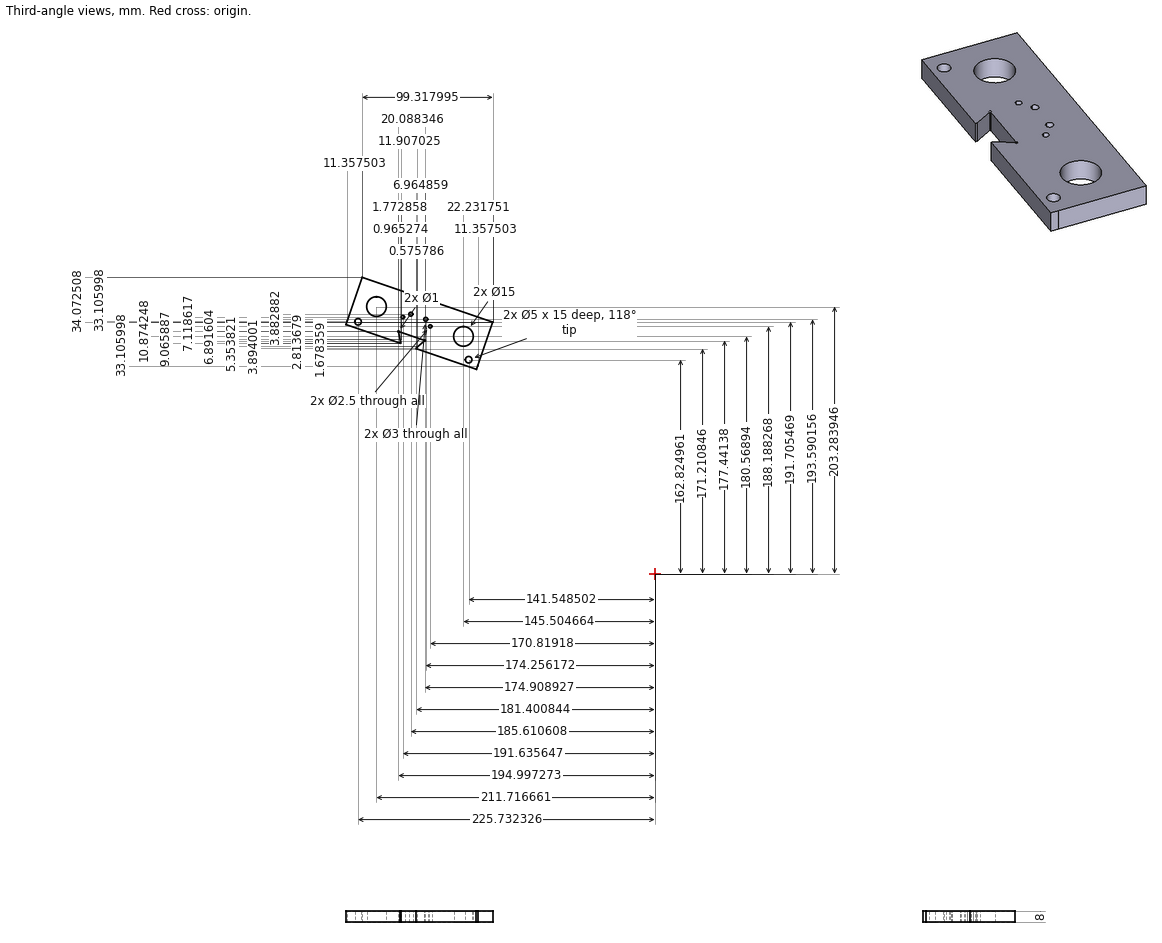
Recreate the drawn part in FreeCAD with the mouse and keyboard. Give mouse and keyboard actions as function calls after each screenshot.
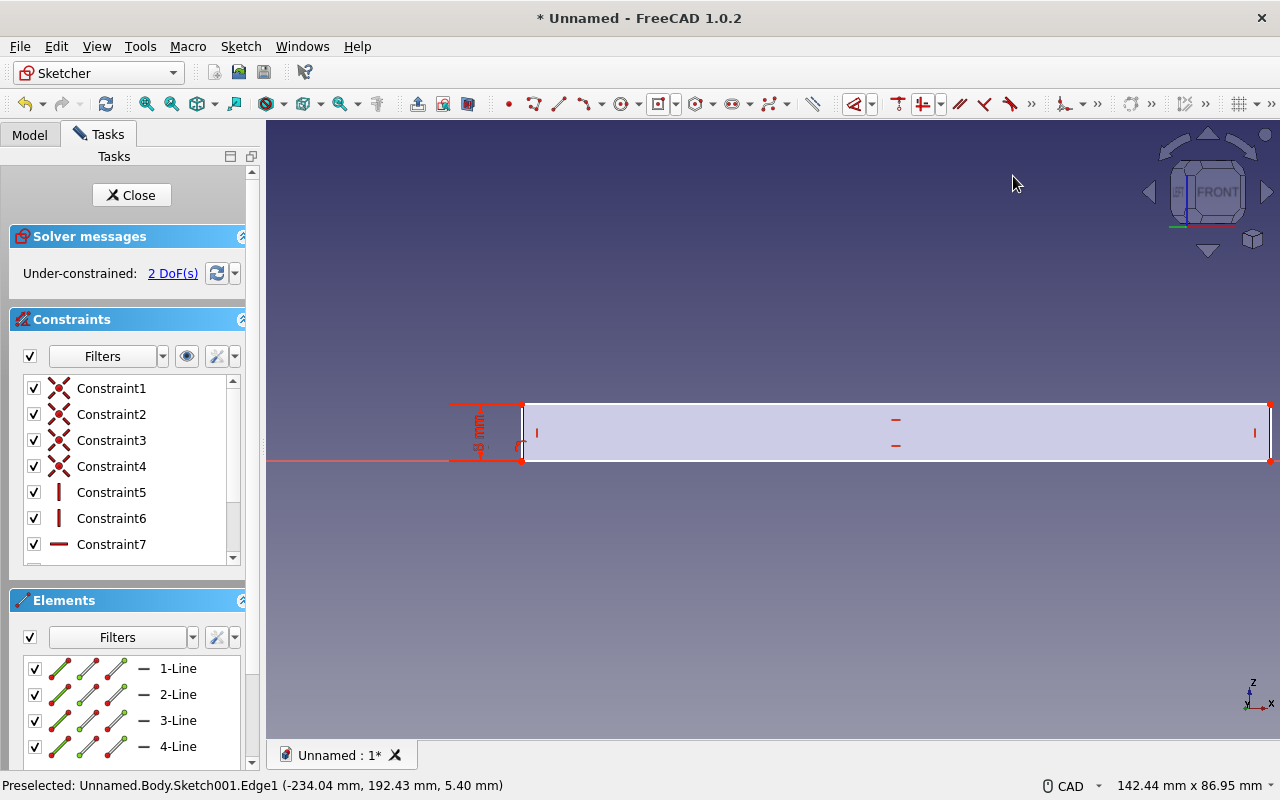
click(747, 461)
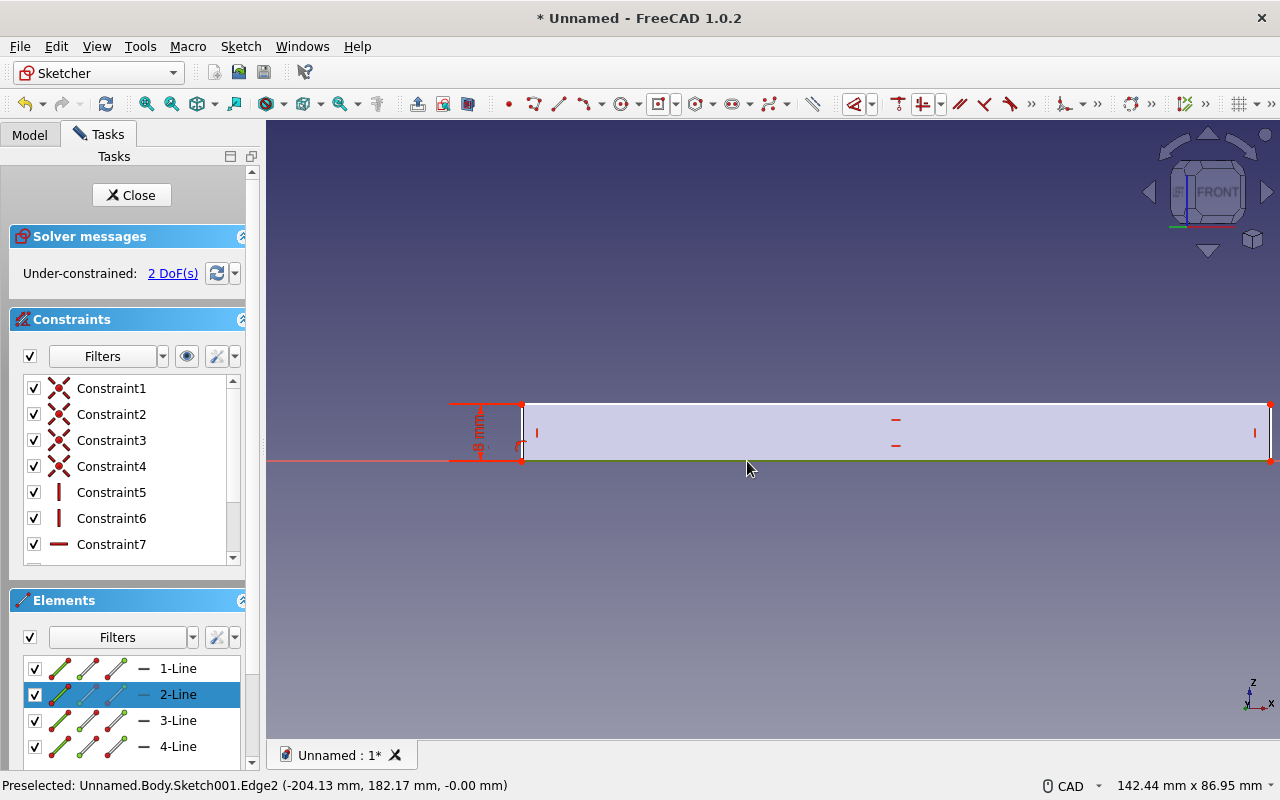
click(872, 104)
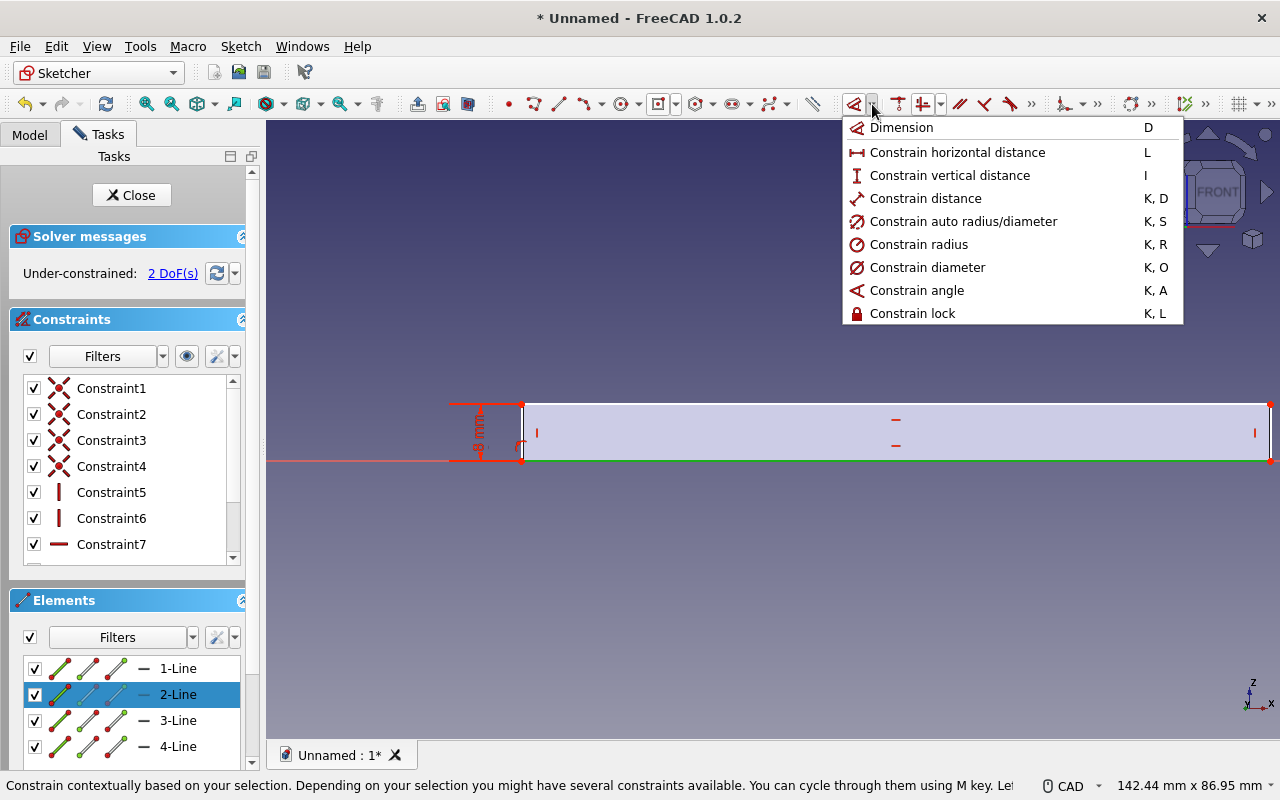
click(1013, 152)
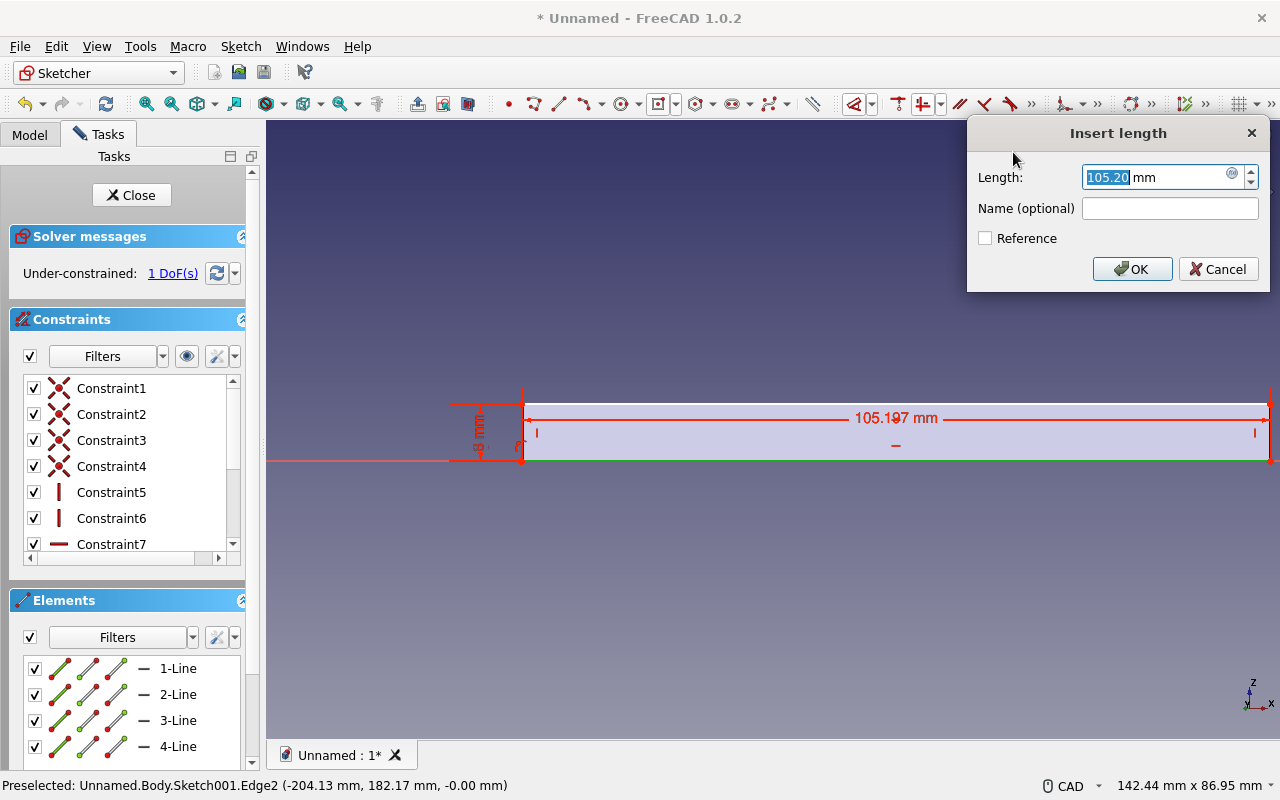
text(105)
key(Return)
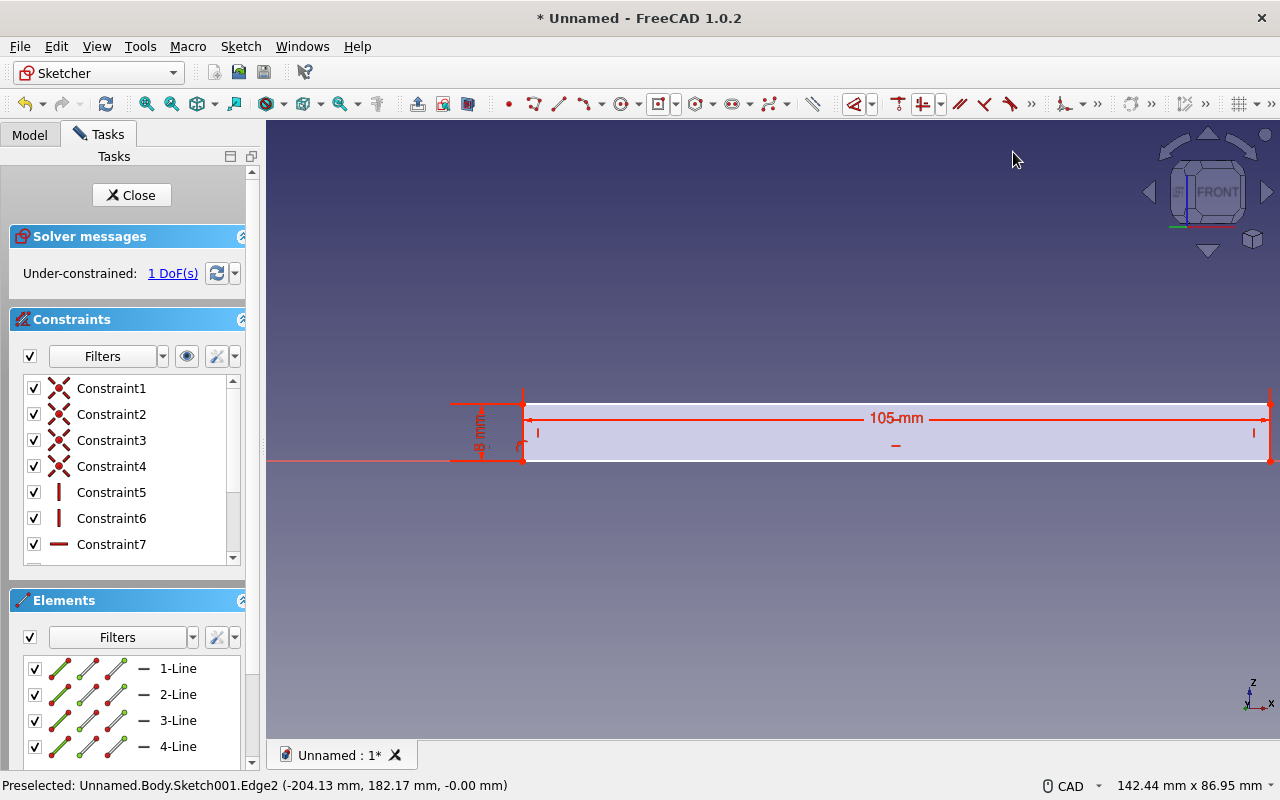
click(523, 404)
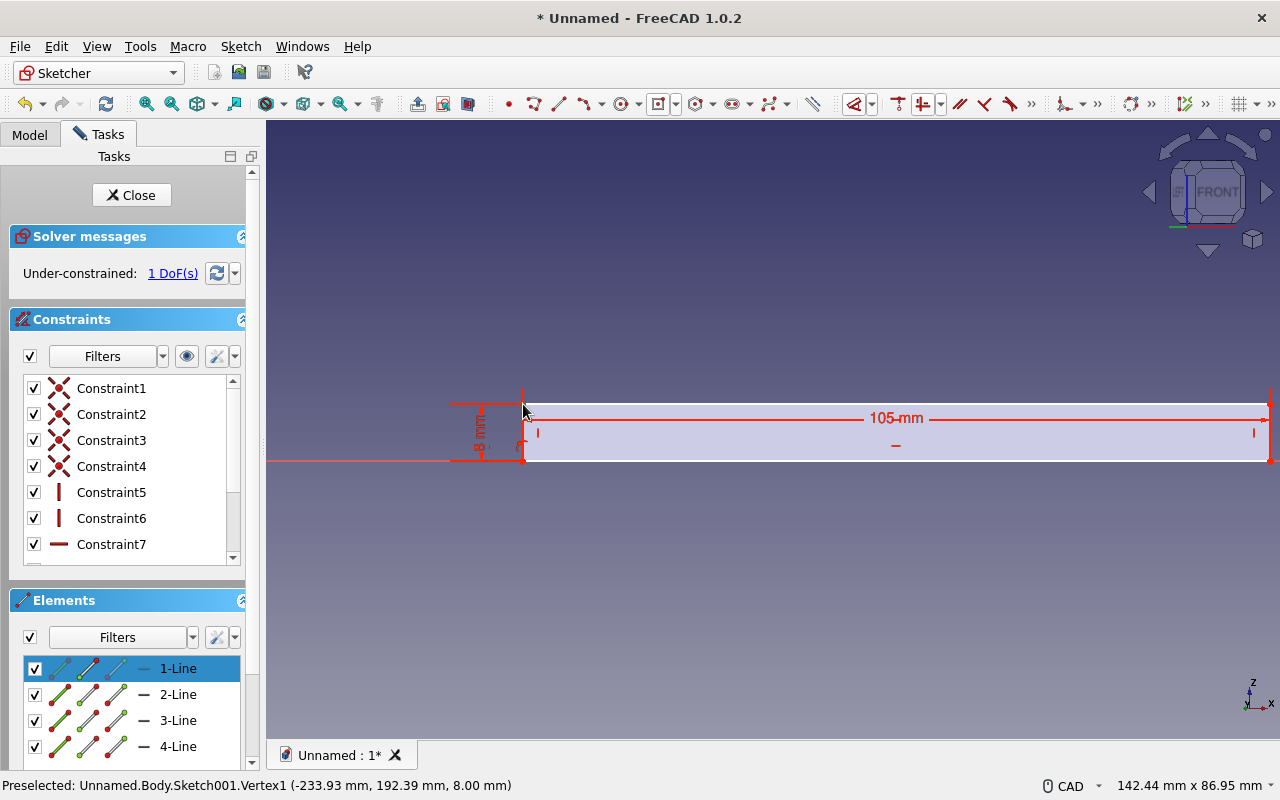
key(l)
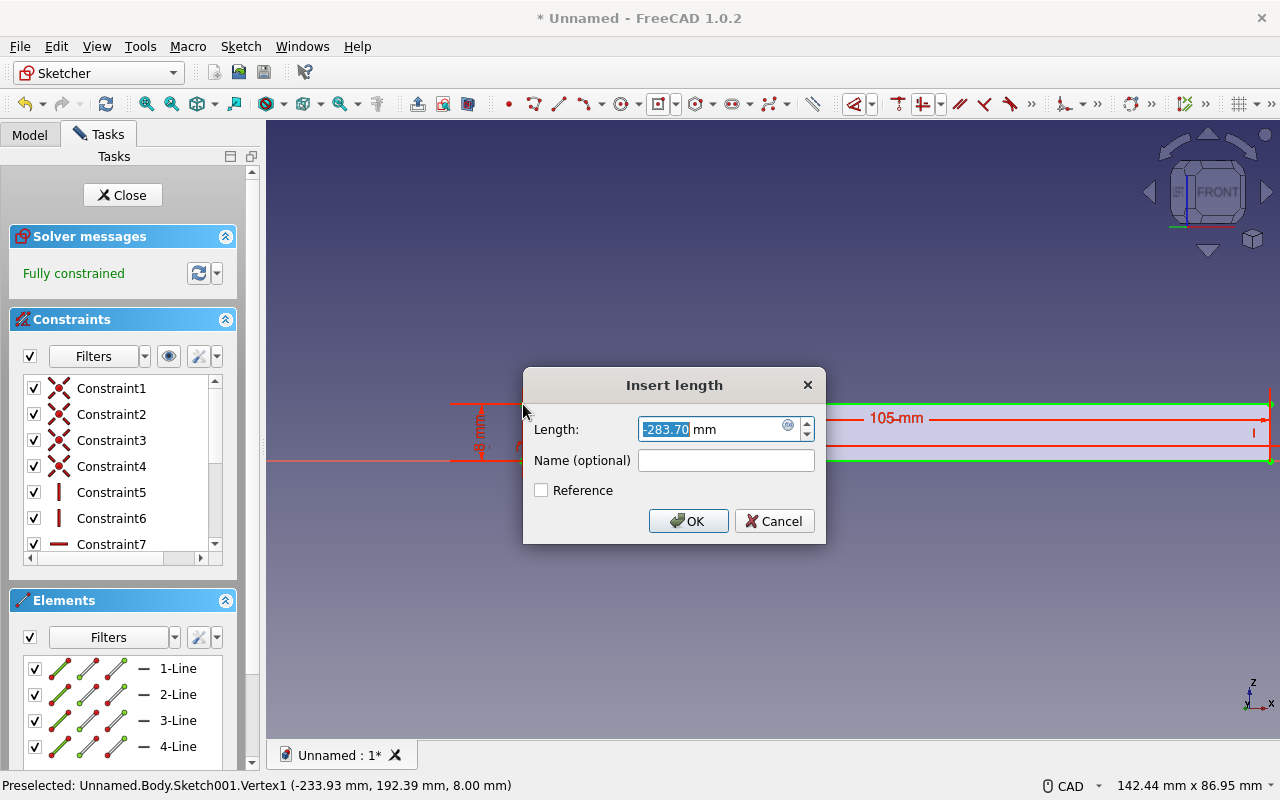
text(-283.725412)
key(Return)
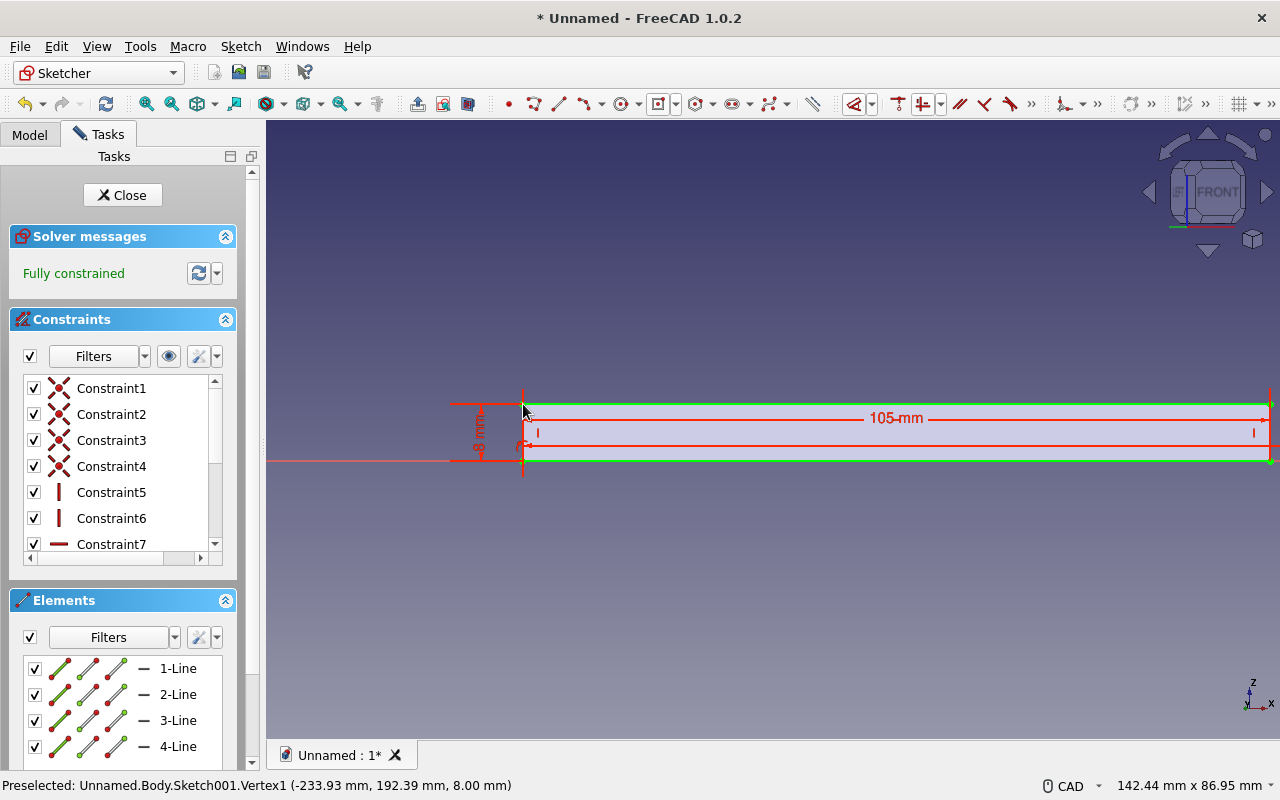
click(123, 195)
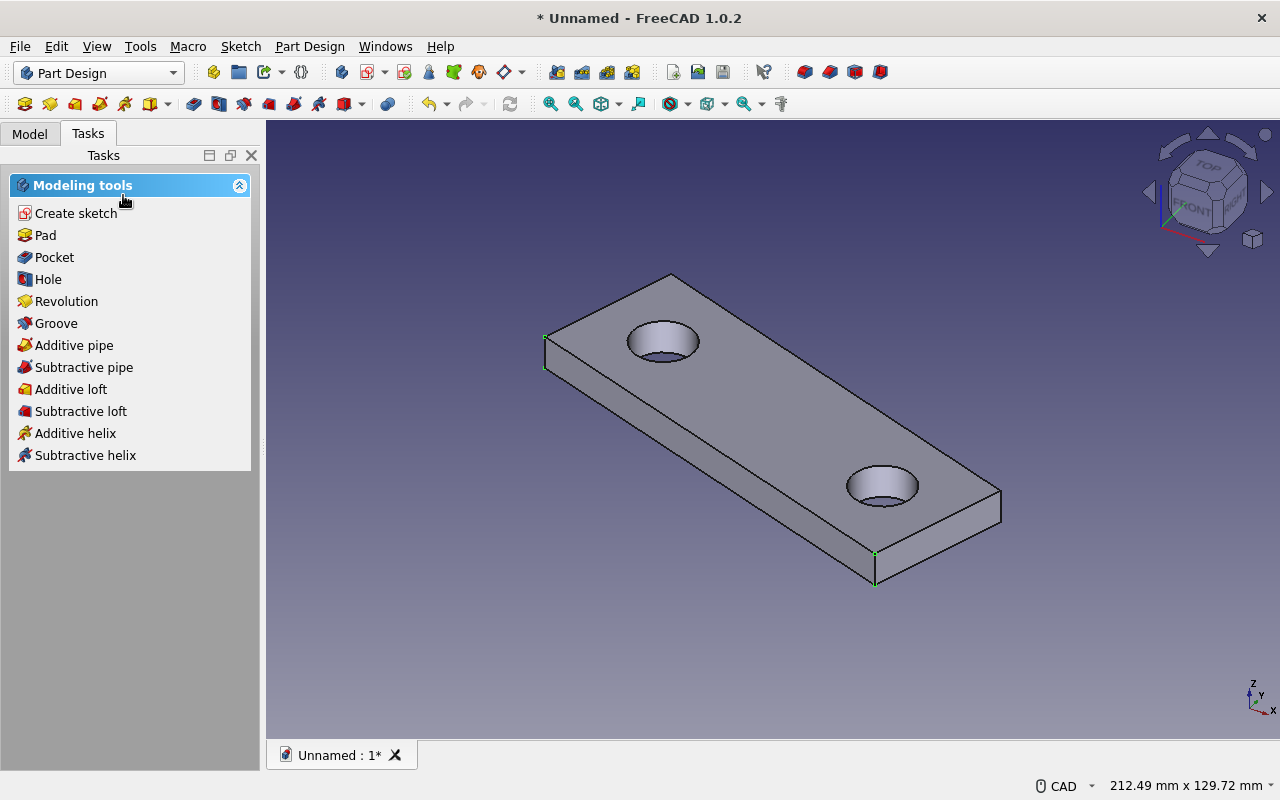
click(25, 104)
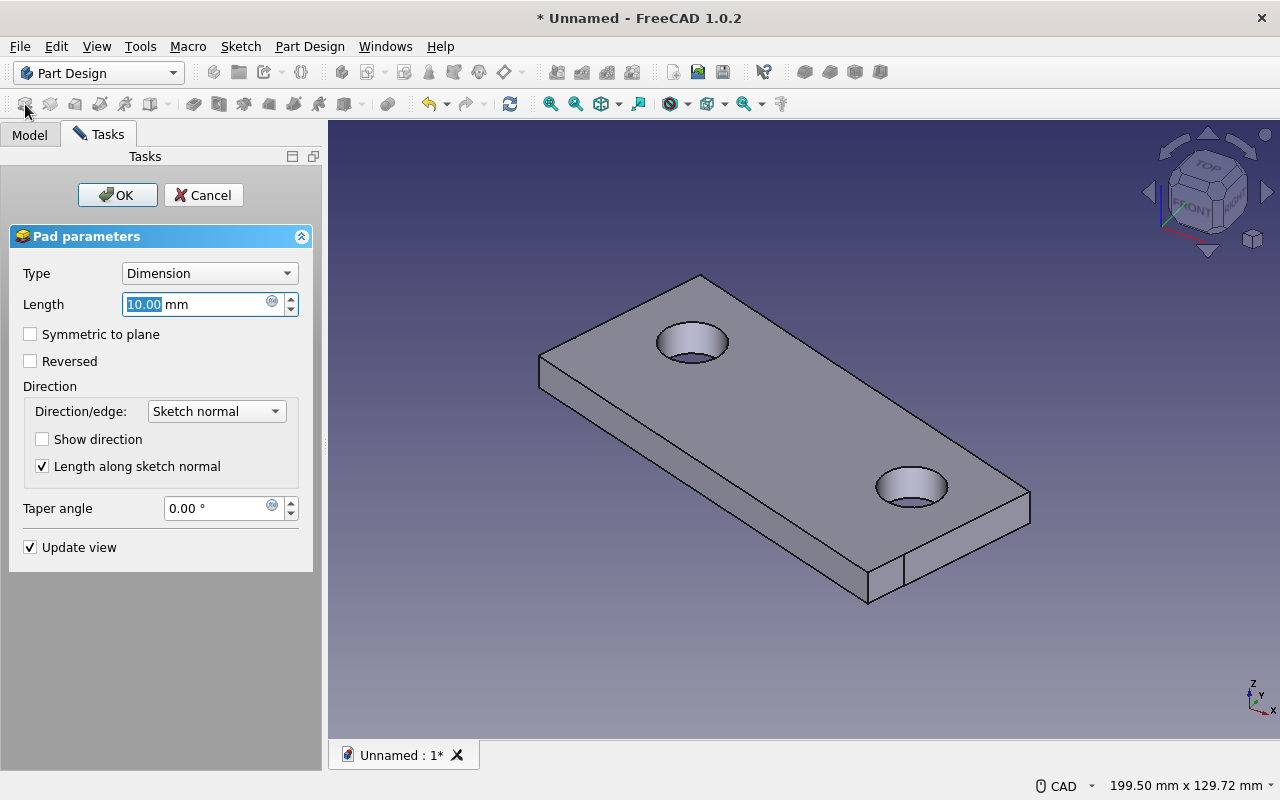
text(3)
key(Tab)